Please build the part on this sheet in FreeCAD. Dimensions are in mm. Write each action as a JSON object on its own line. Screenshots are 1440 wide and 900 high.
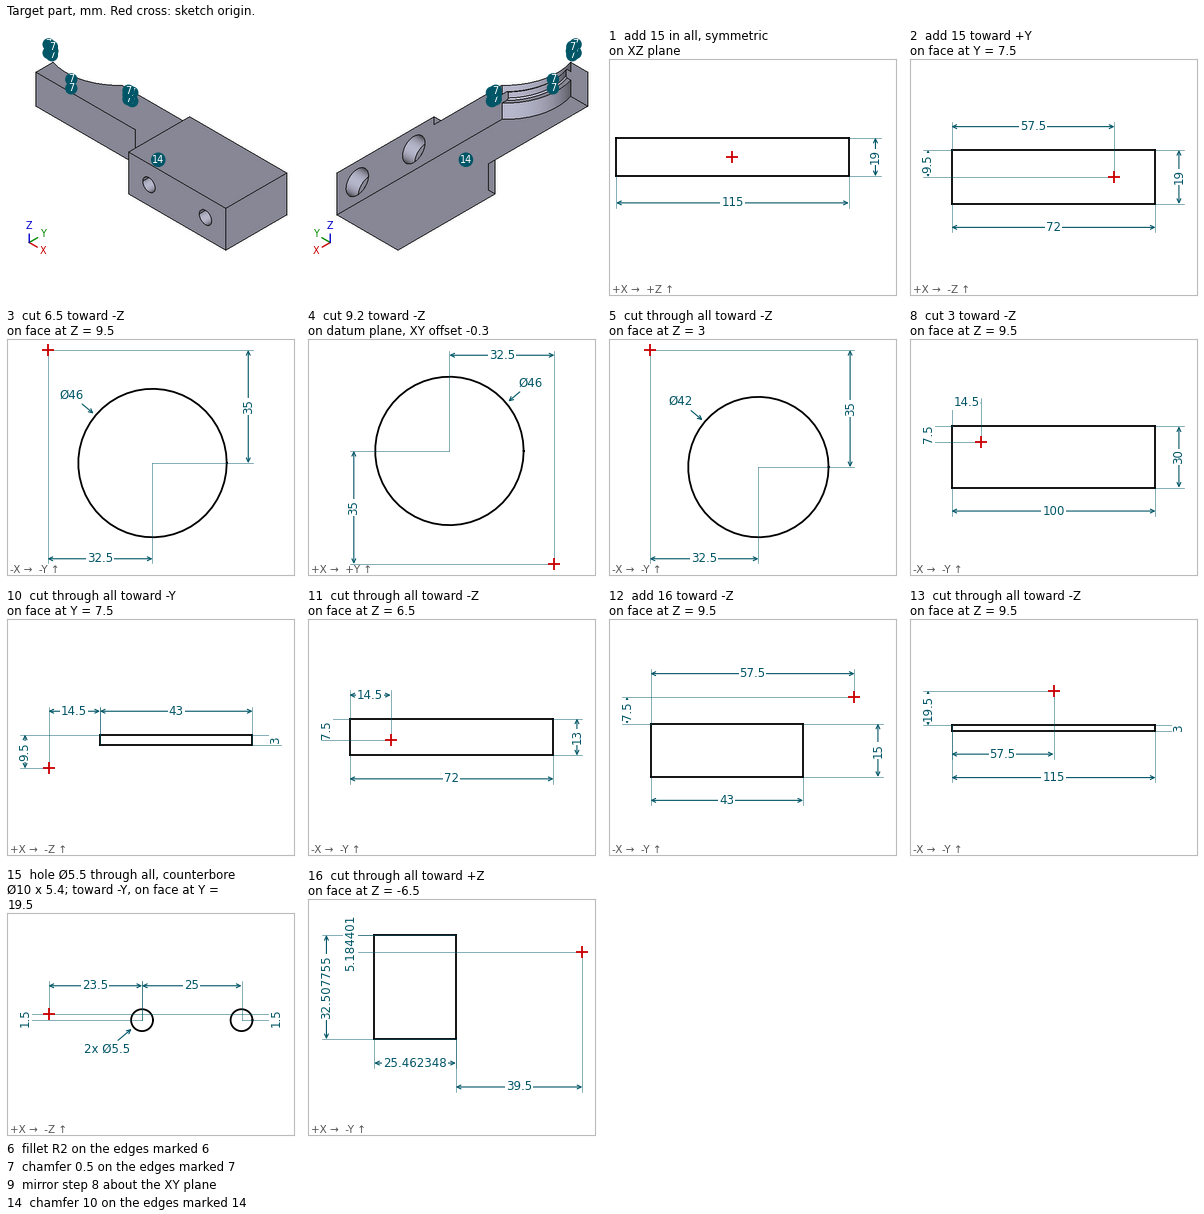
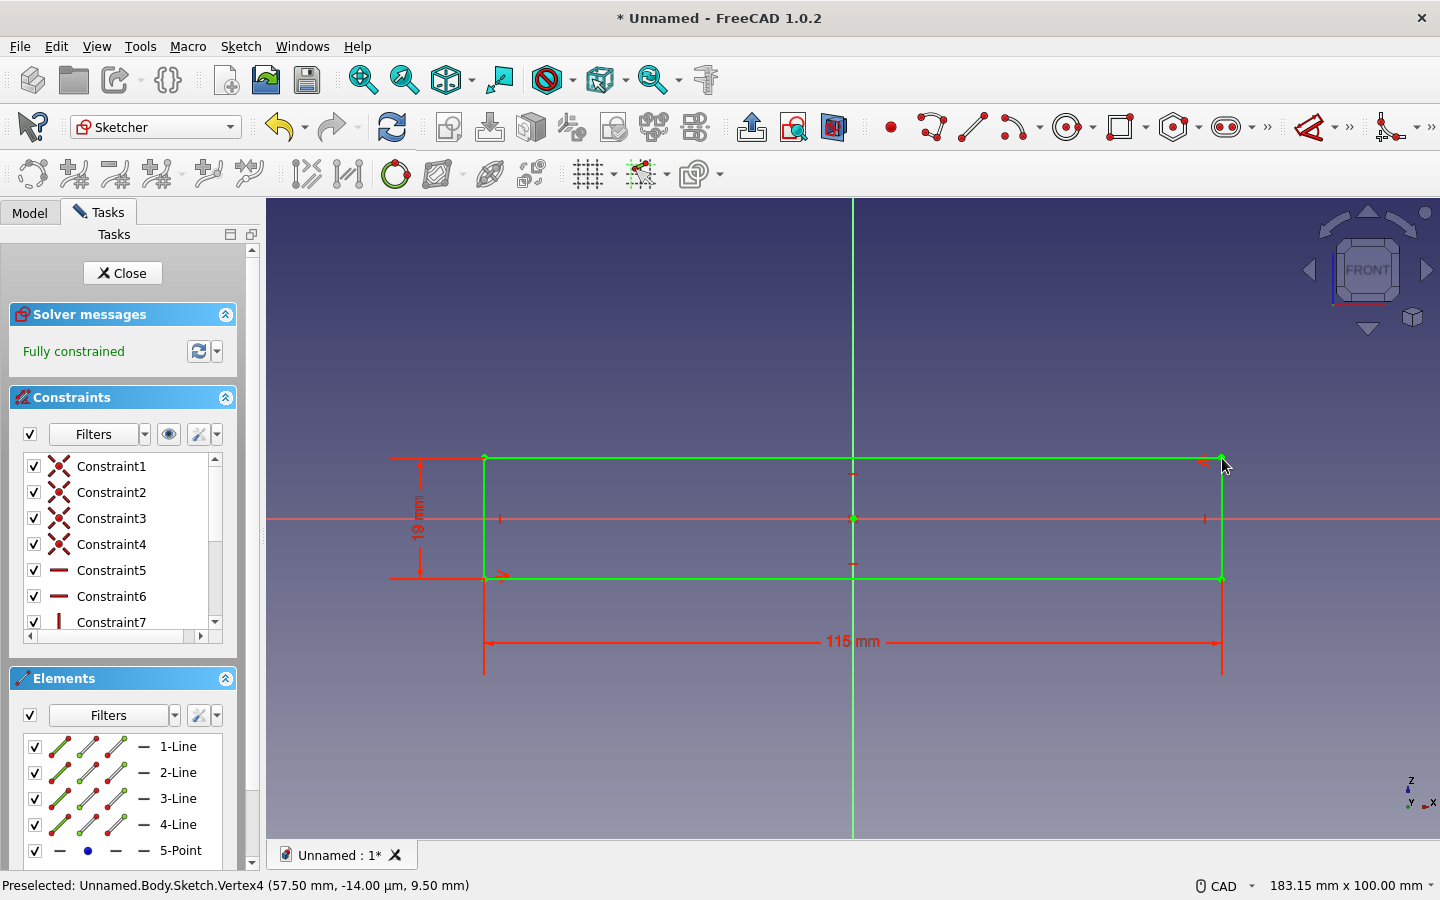
{"action": "left_click", "coordinate": [123, 273]}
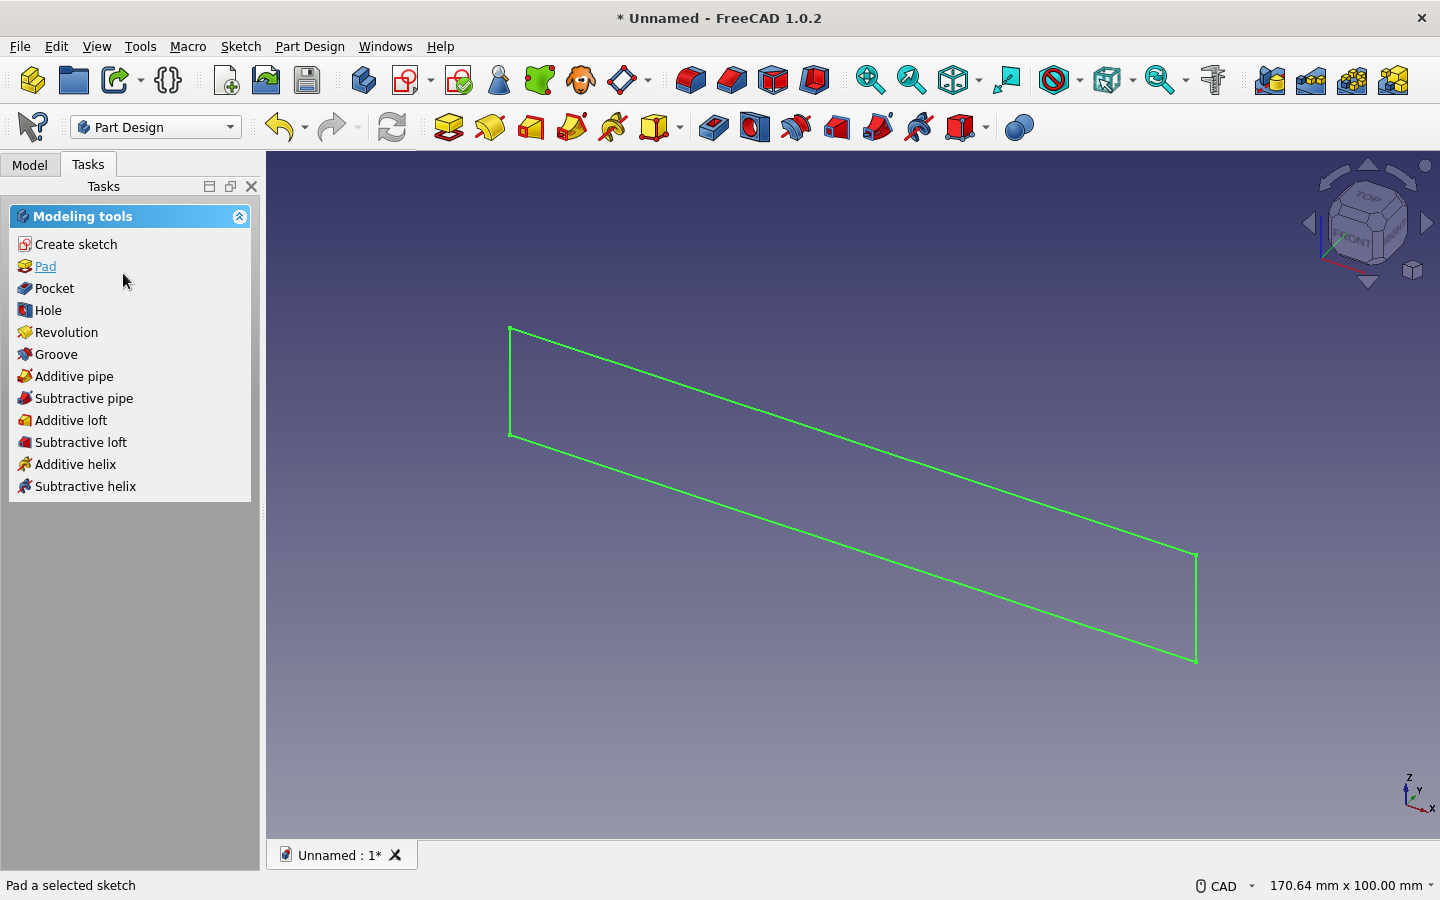
{"action": "left_click", "coordinate": [449, 128]}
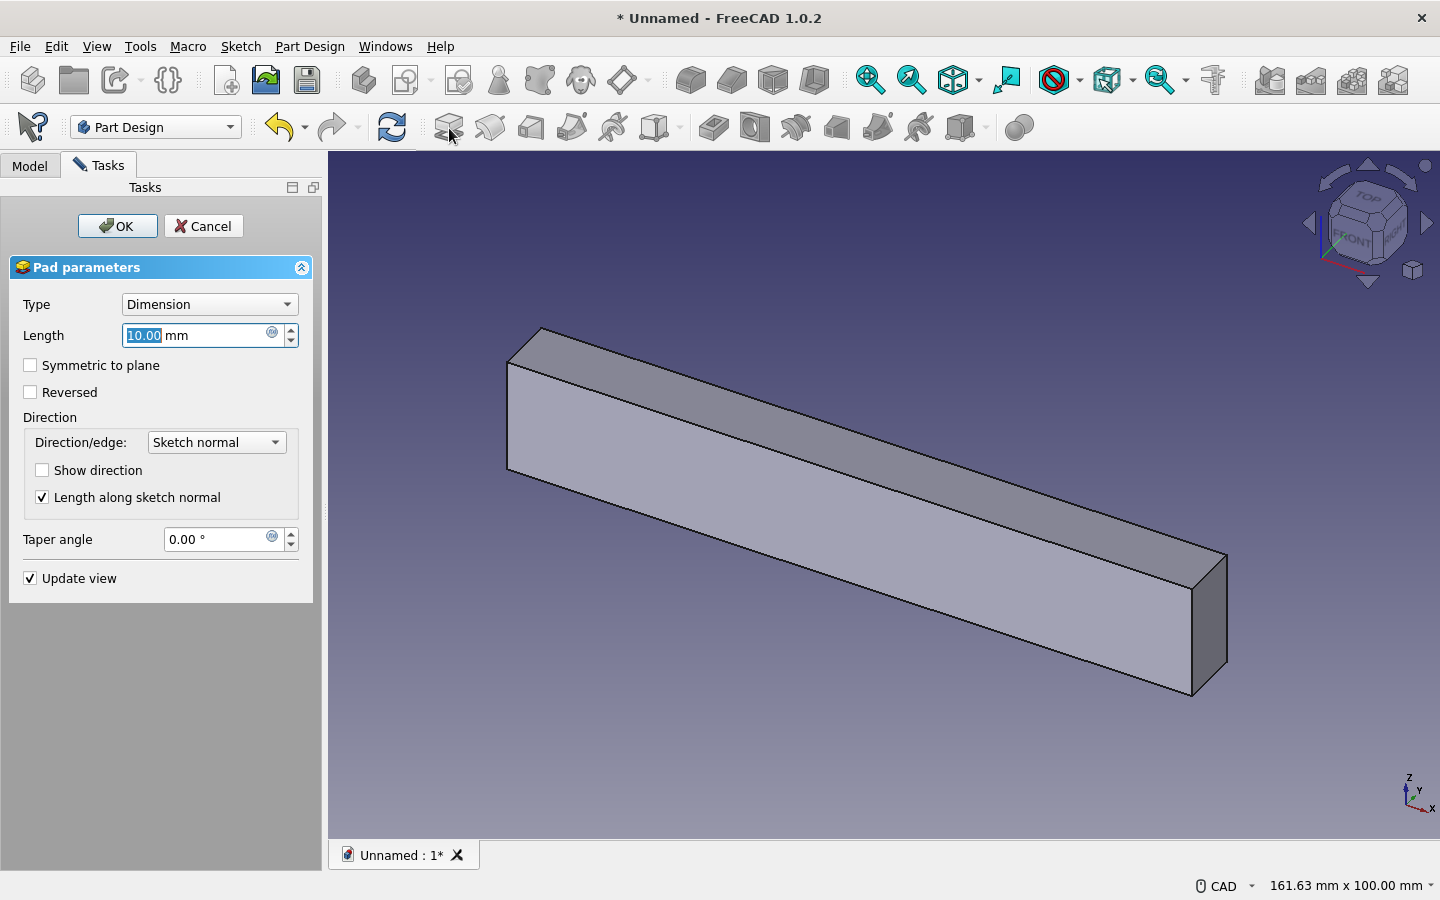
{"action": "type", "text": "15"}
{"action": "key", "text": "Tab"}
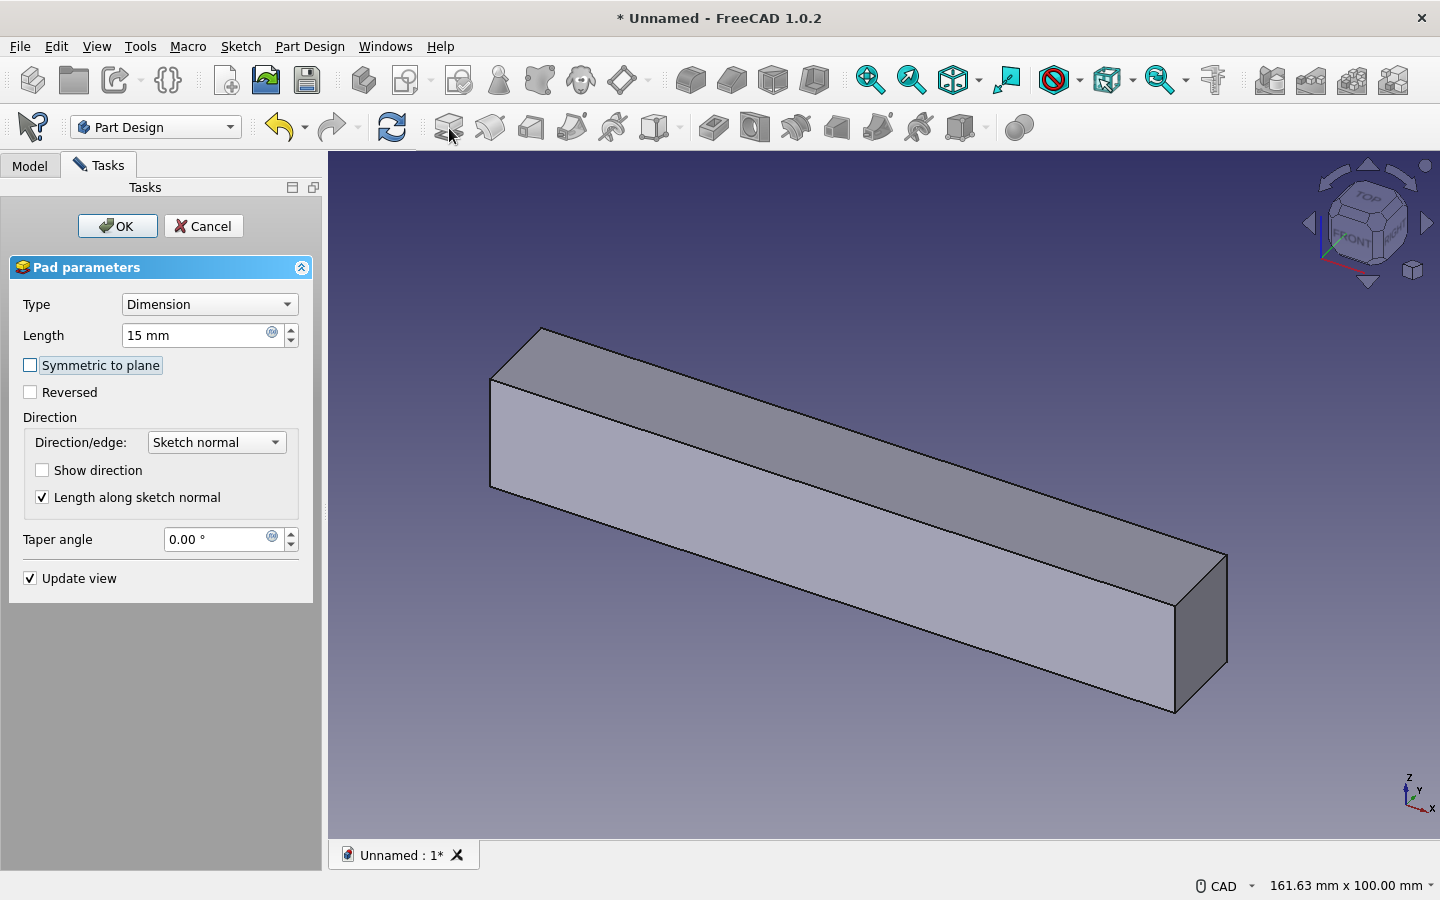
{"action": "left_click", "coordinate": [31, 365]}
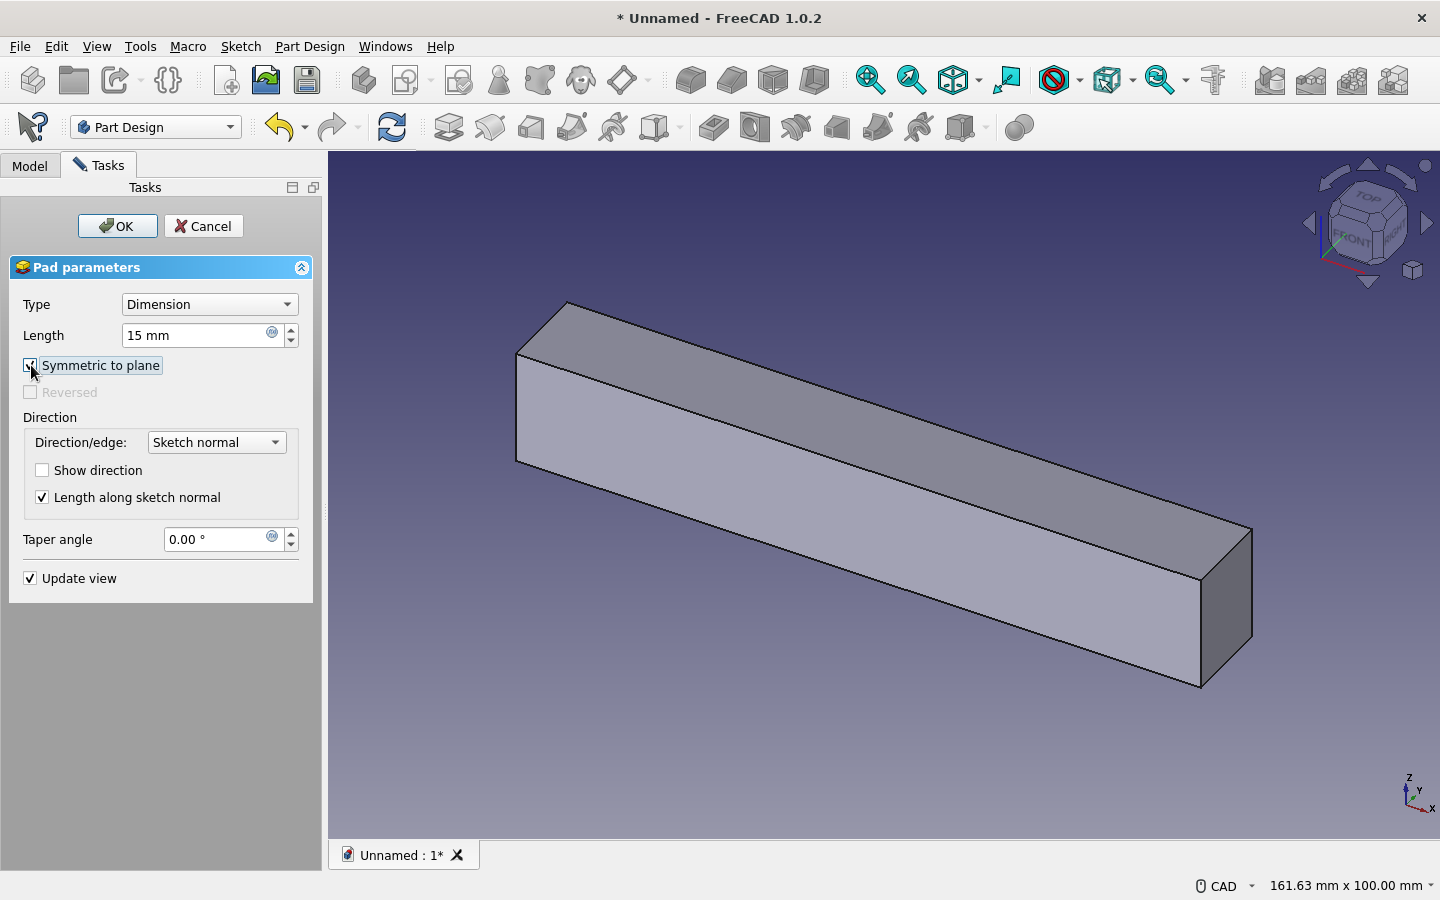
{"action": "left_click", "coordinate": [118, 226]}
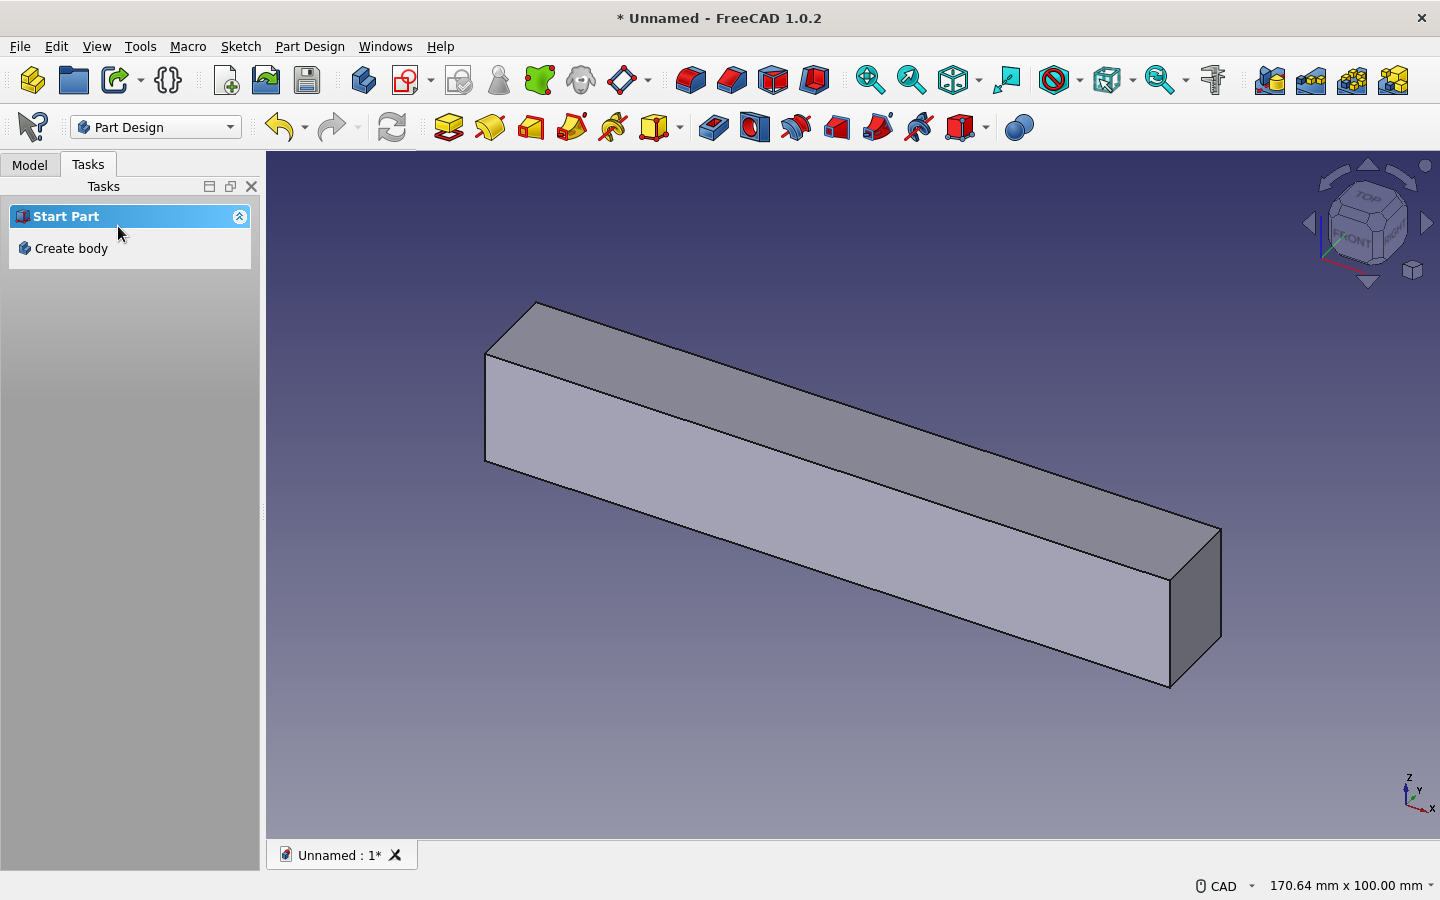
{"action": "key", "text": "4"}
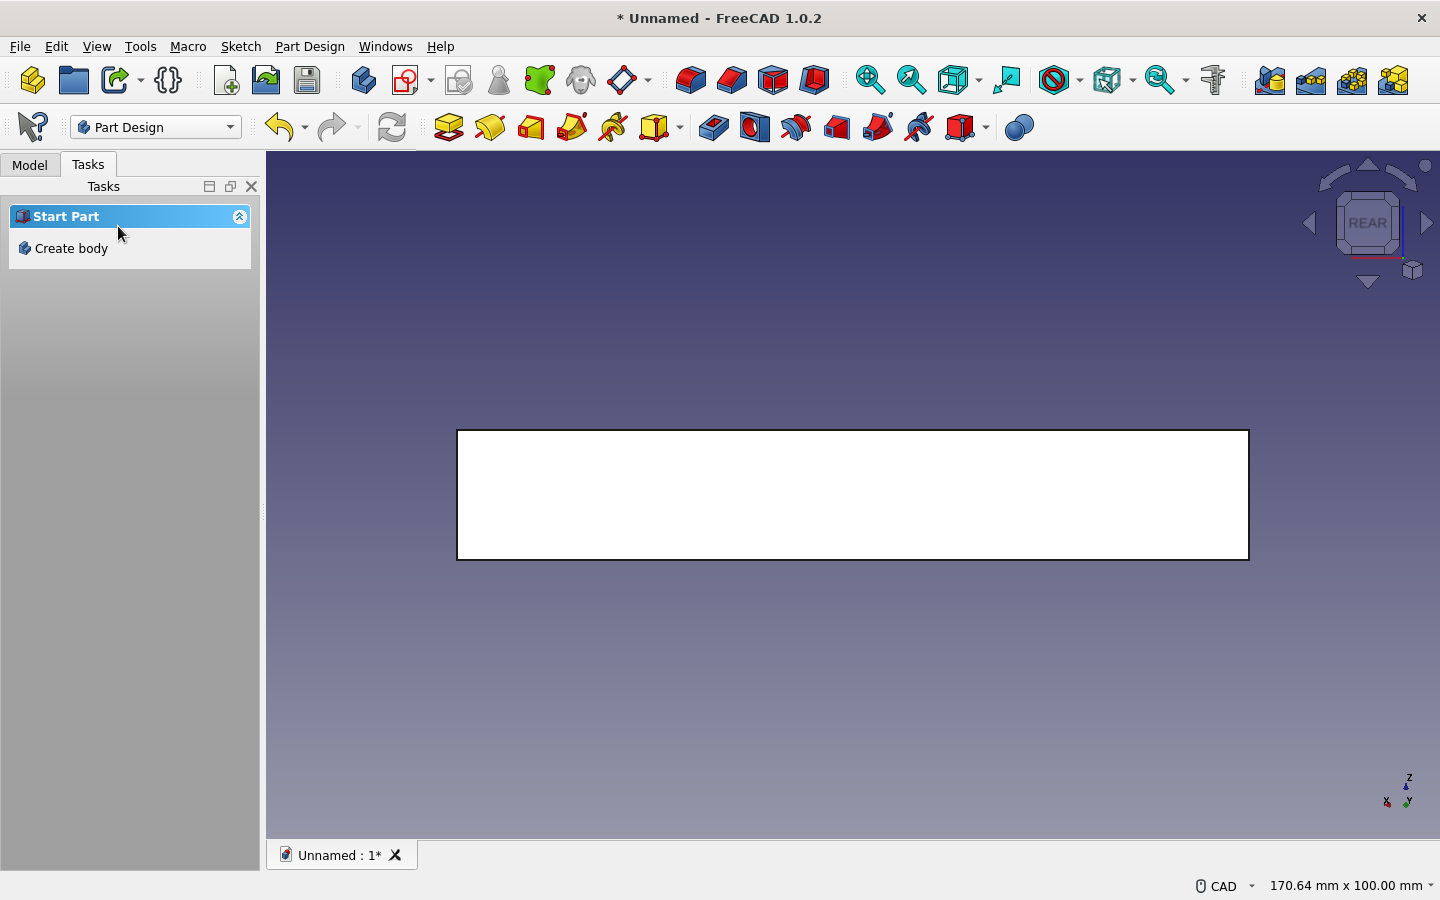
{"action": "left_click", "coordinate": [627, 494]}